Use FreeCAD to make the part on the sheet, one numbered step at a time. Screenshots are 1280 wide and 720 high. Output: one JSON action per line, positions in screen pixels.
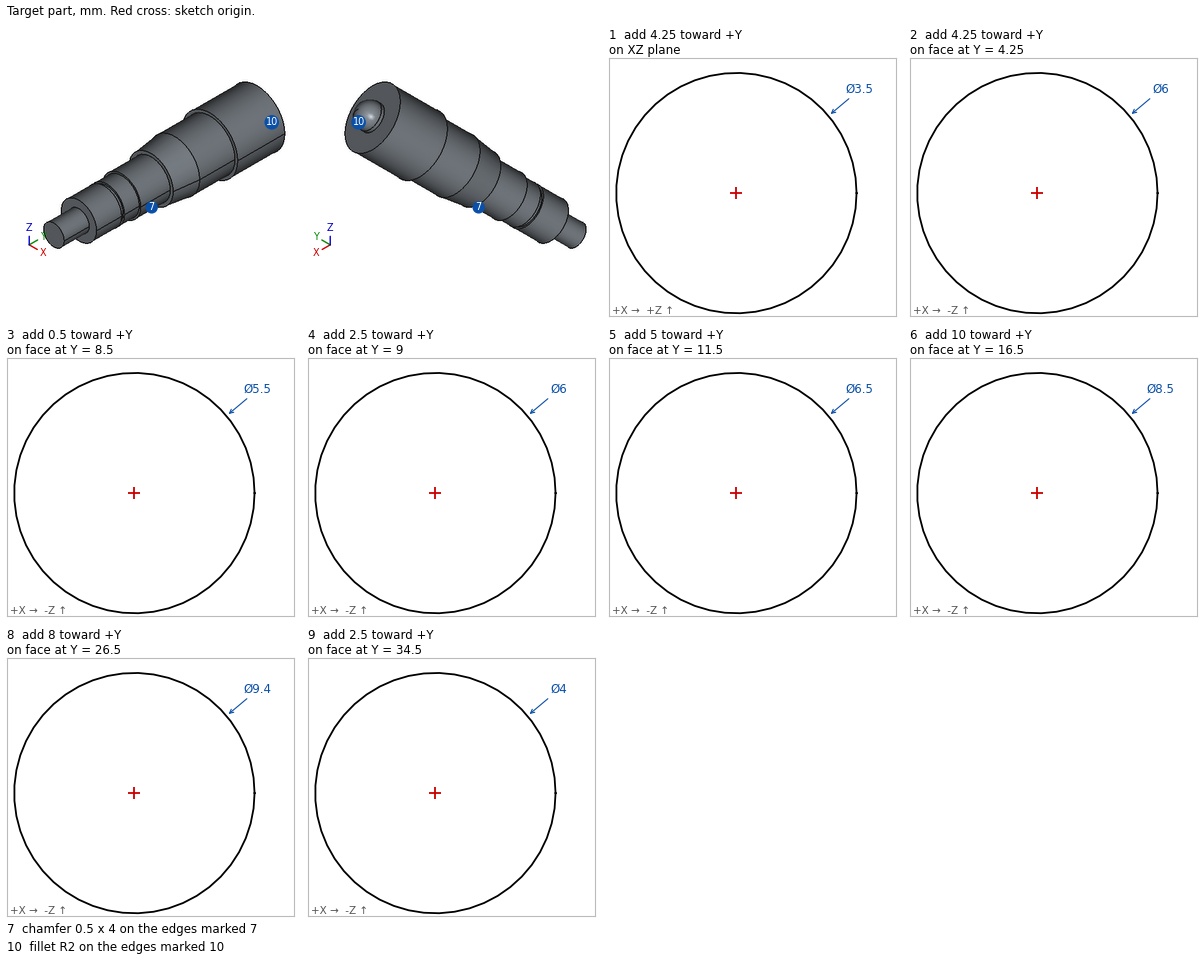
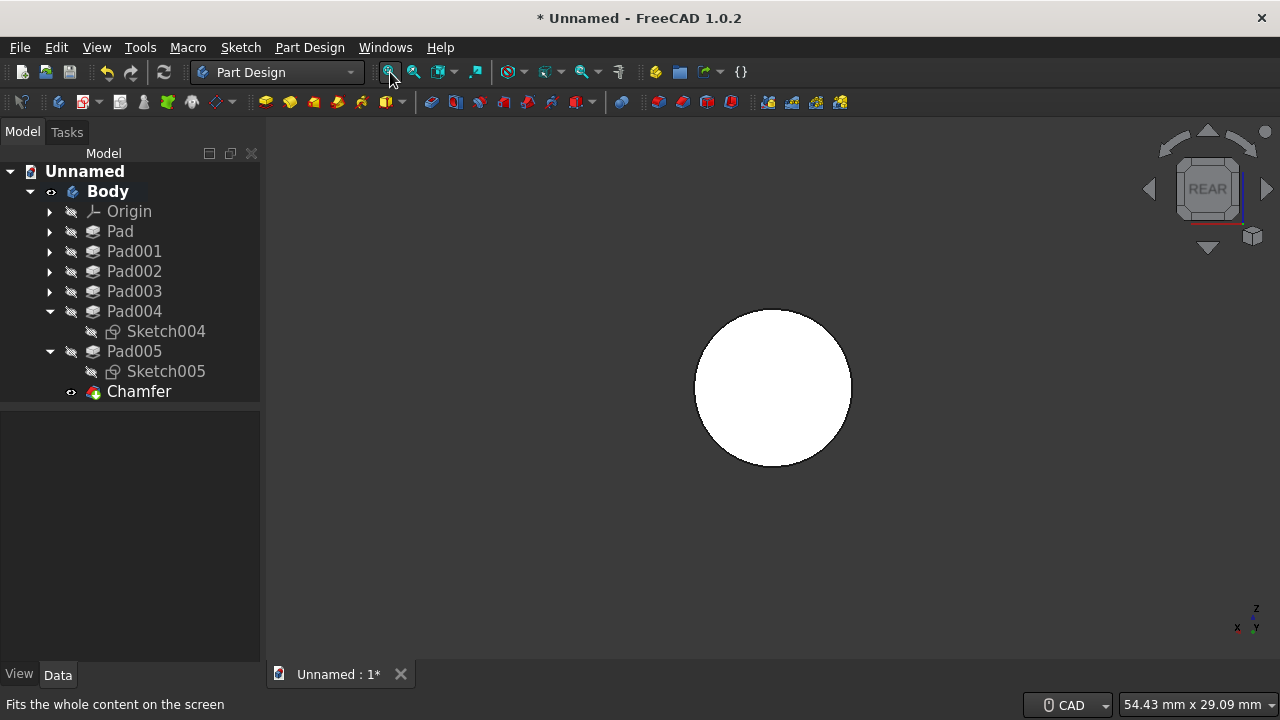
{"action": "left_click", "coordinate": [773, 387]}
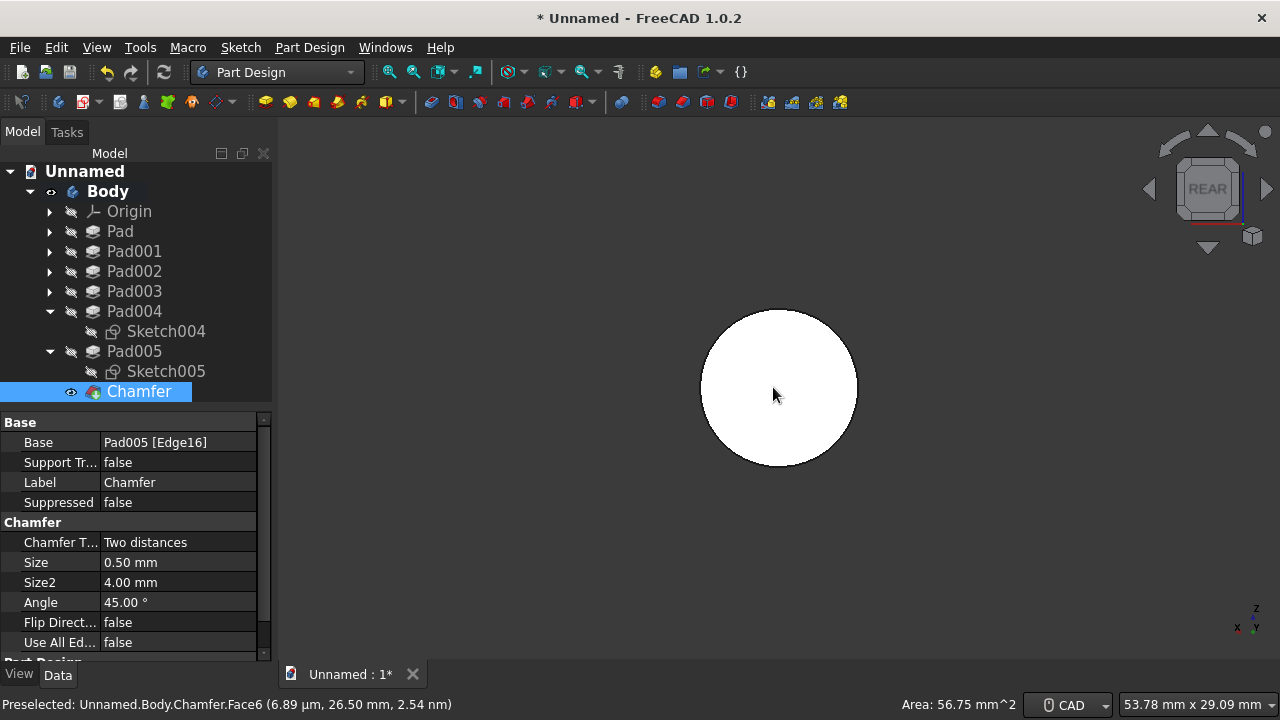
{"action": "left_click", "coordinate": [84, 102]}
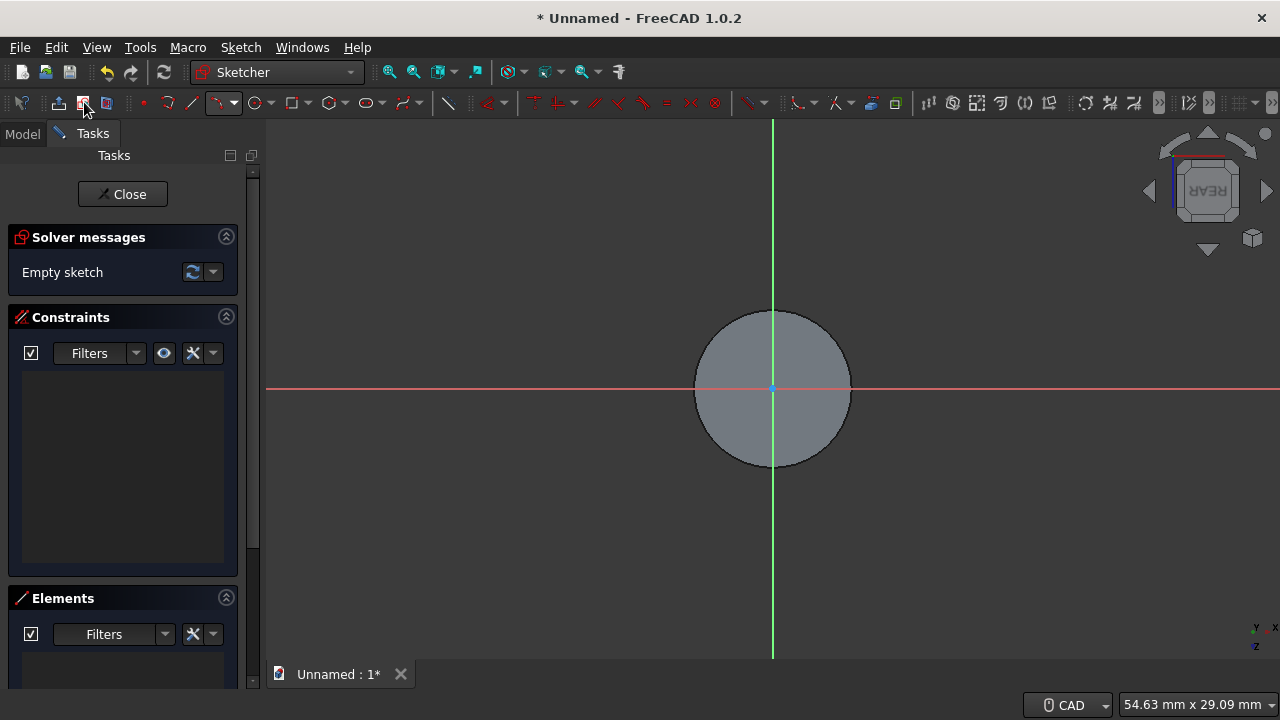
{"action": "scroll", "coordinate": [856, 389], "scroll_direction": "up", "scroll_amount": 3}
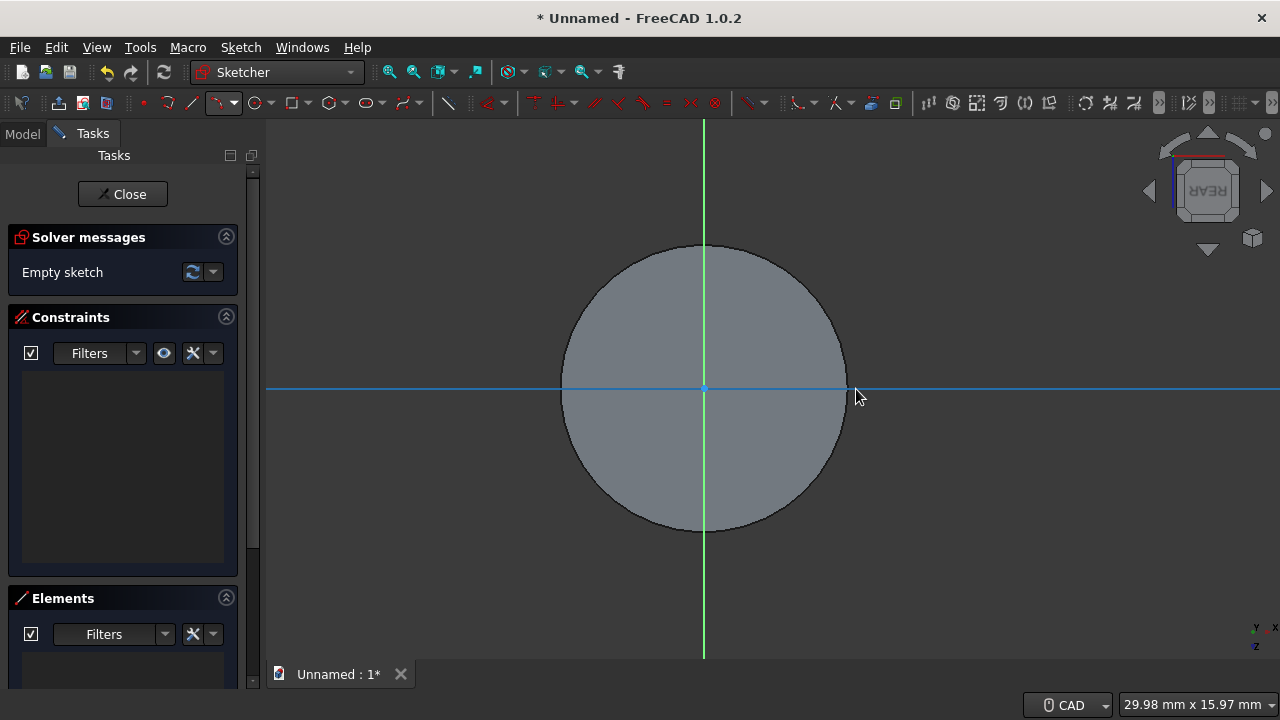
{"action": "key", "text": "g c"}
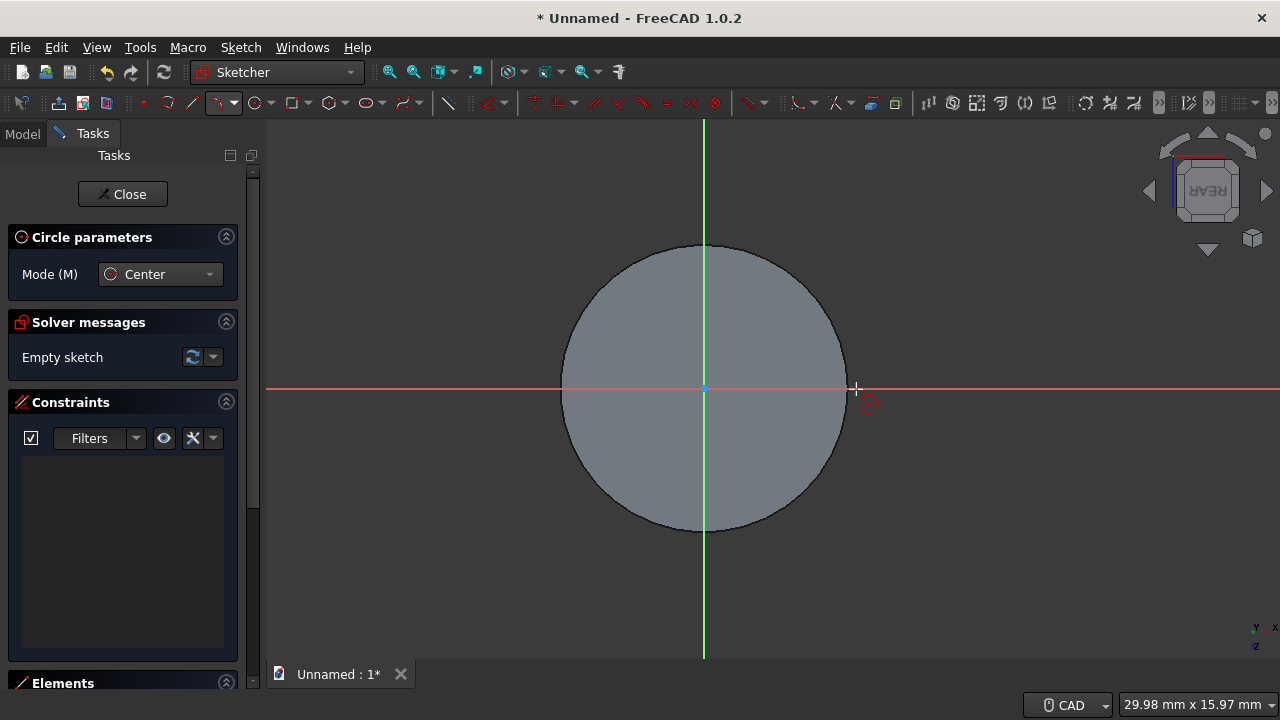
{"action": "left_click", "coordinate": [704, 389]}
{"action": "mouse_move", "coordinate": [816, 276]}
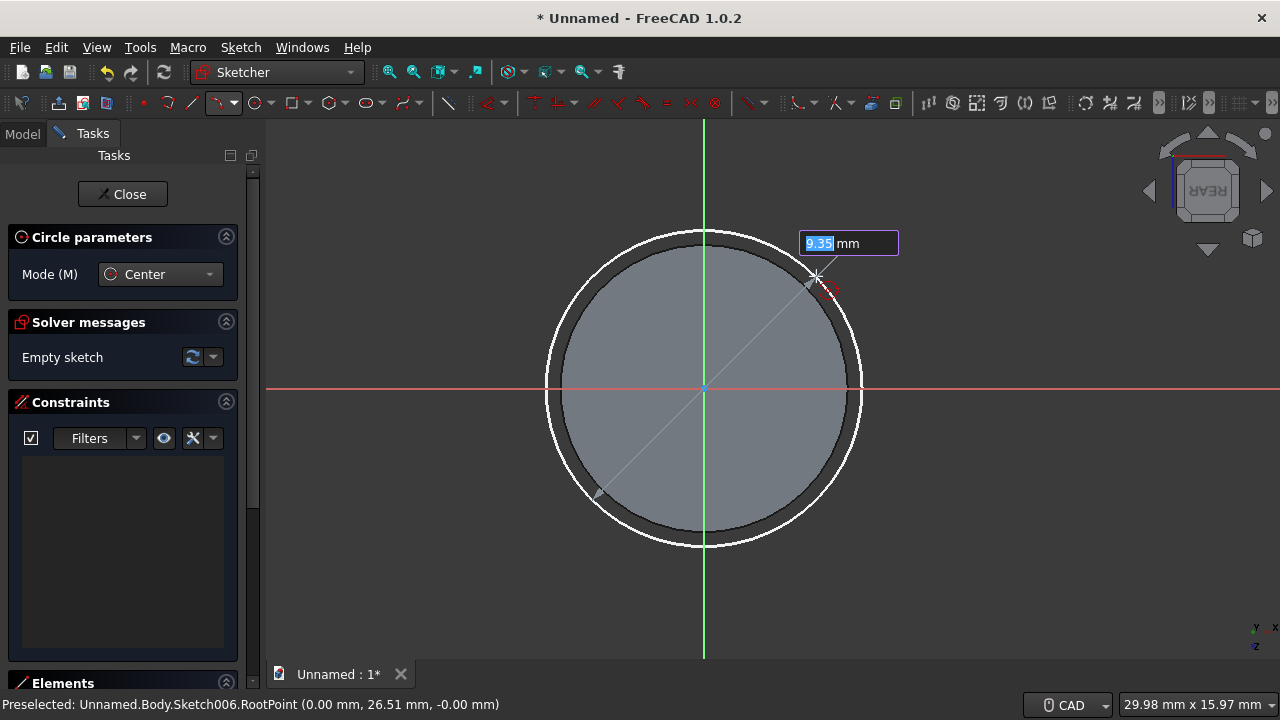
{"action": "type", "text": "9.4"}
{"action": "key", "text": "Return"}
{"action": "key", "text": "Escape"}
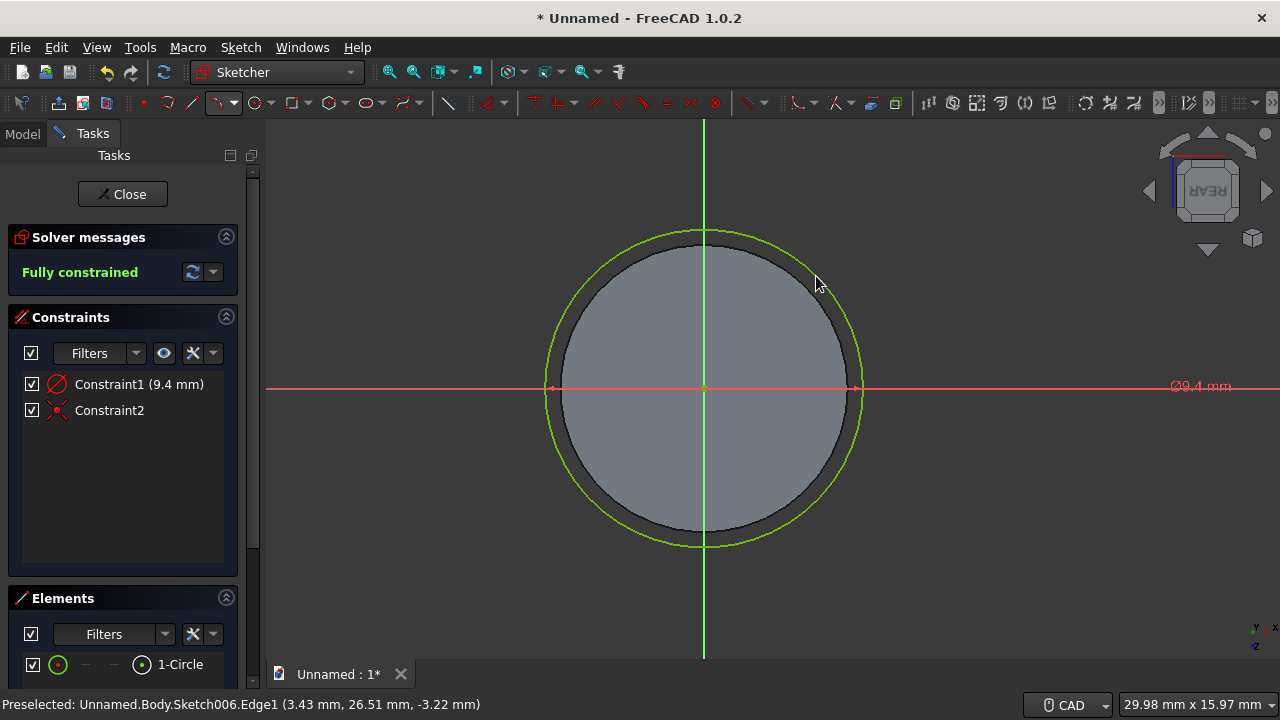
{"action": "left_click", "coordinate": [123, 194]}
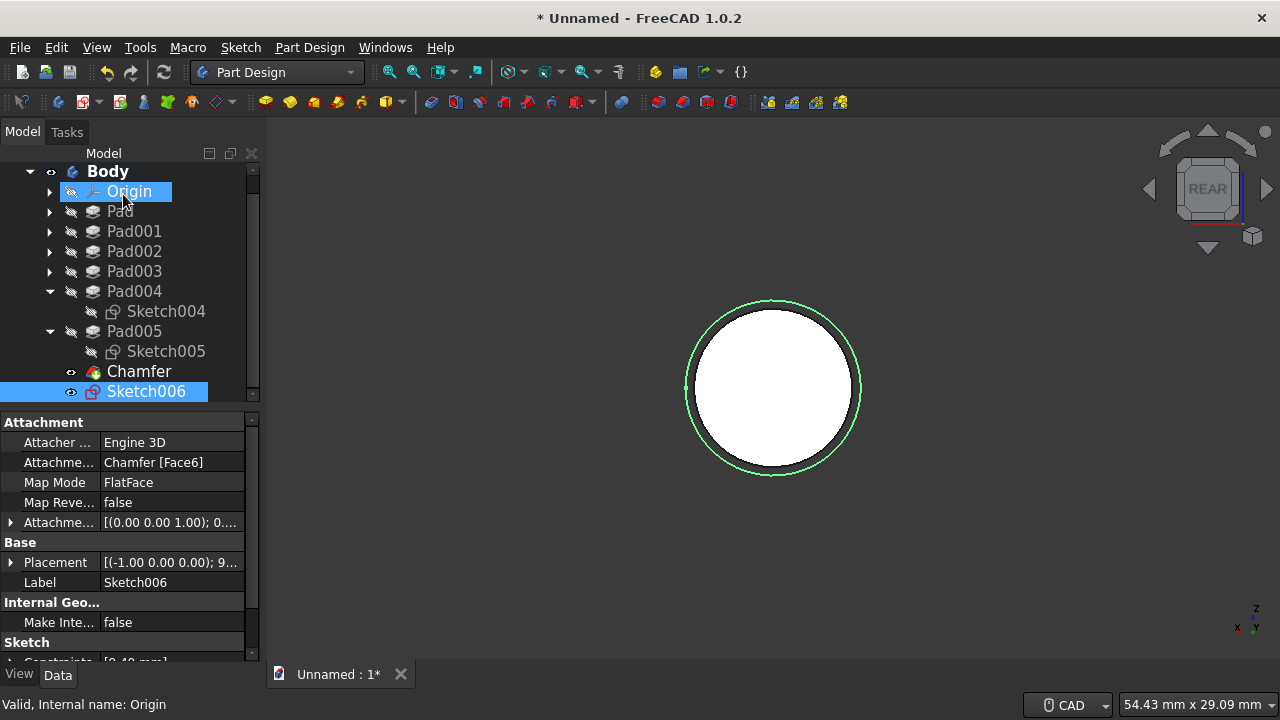
{"action": "left_click", "coordinate": [266, 102]}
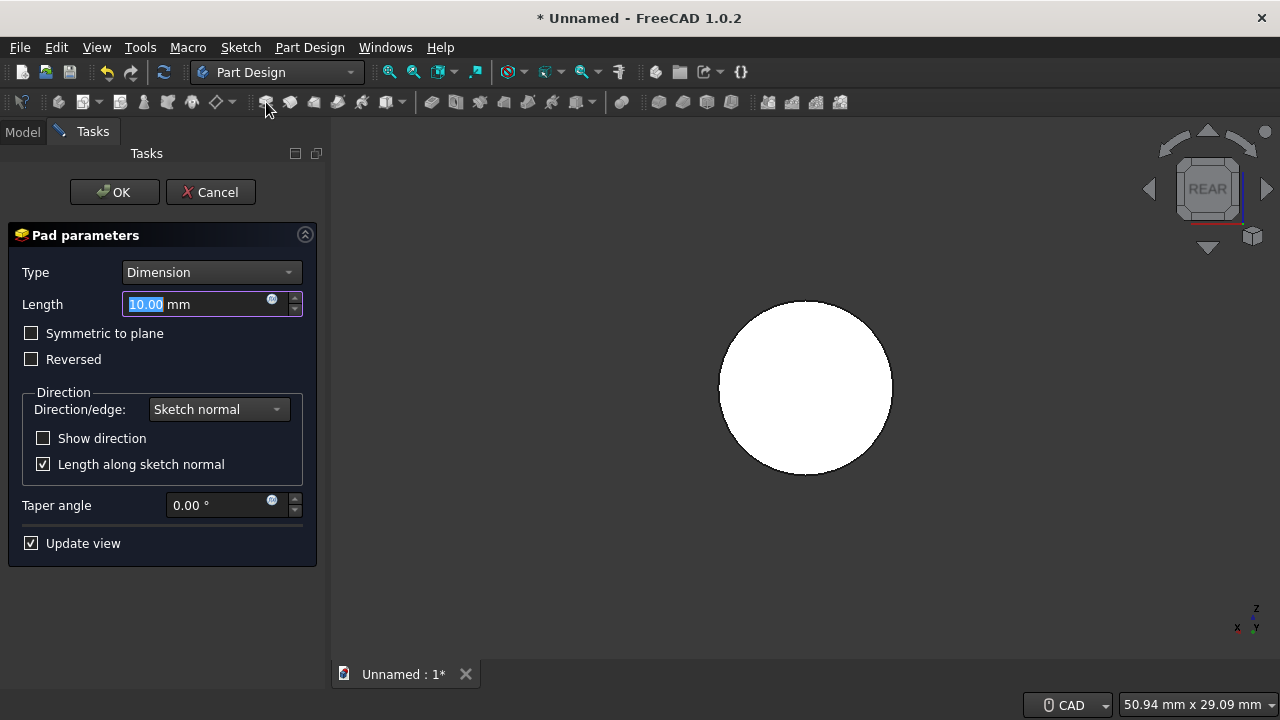
{"action": "type", "text": "8"}
{"action": "key", "text": "Tab"}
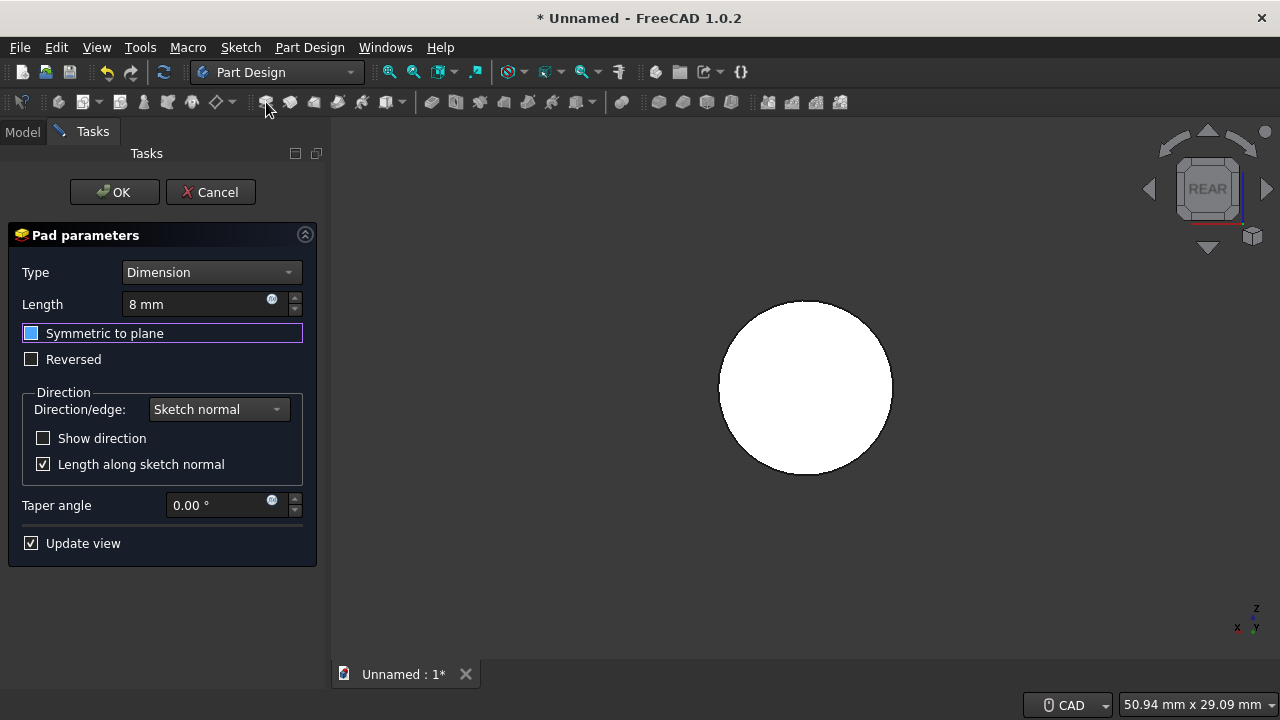
{"action": "left_click", "coordinate": [115, 192]}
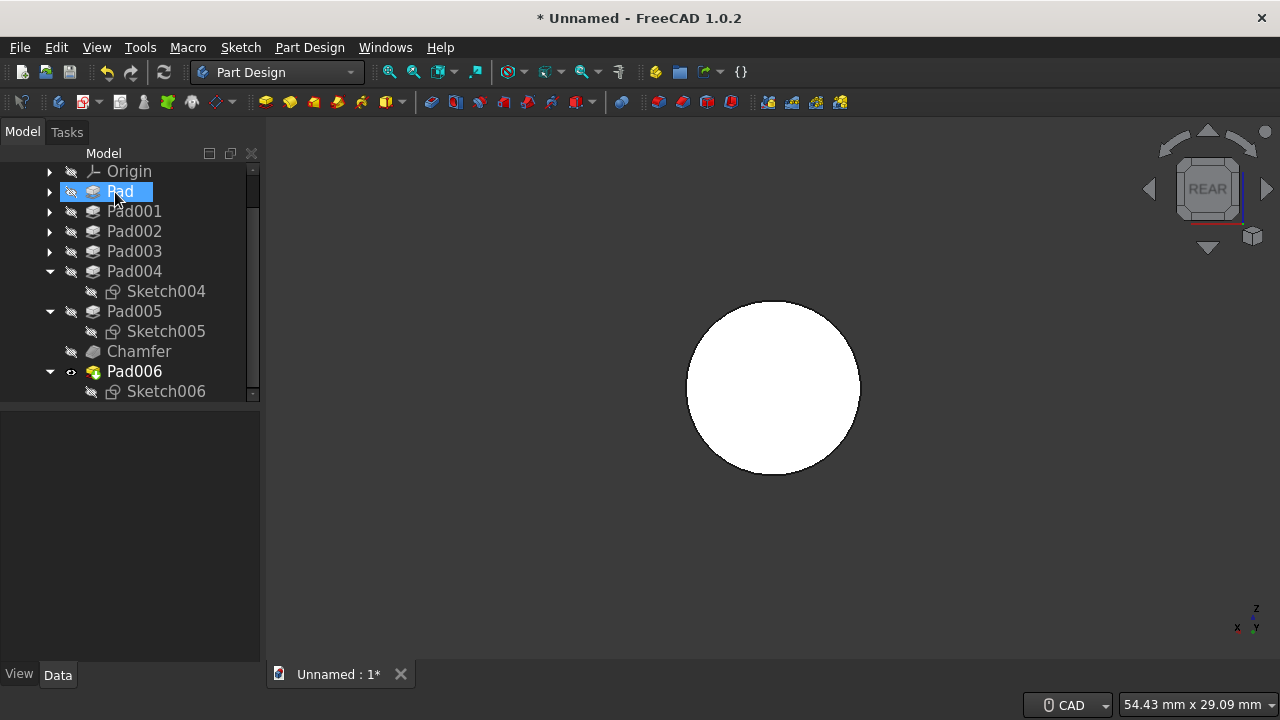
{"action": "left_click", "coordinate": [390, 72]}